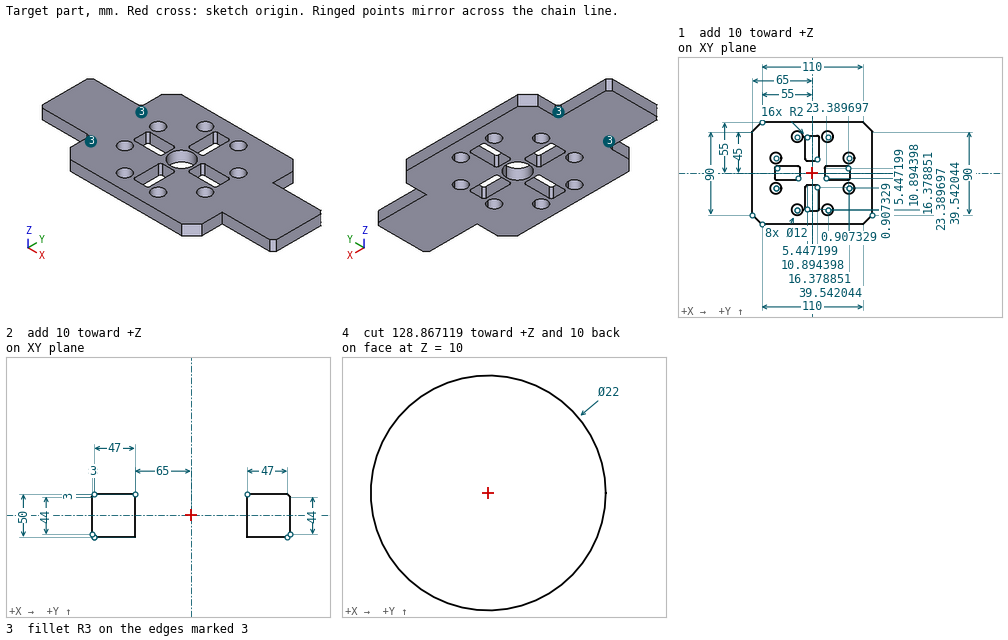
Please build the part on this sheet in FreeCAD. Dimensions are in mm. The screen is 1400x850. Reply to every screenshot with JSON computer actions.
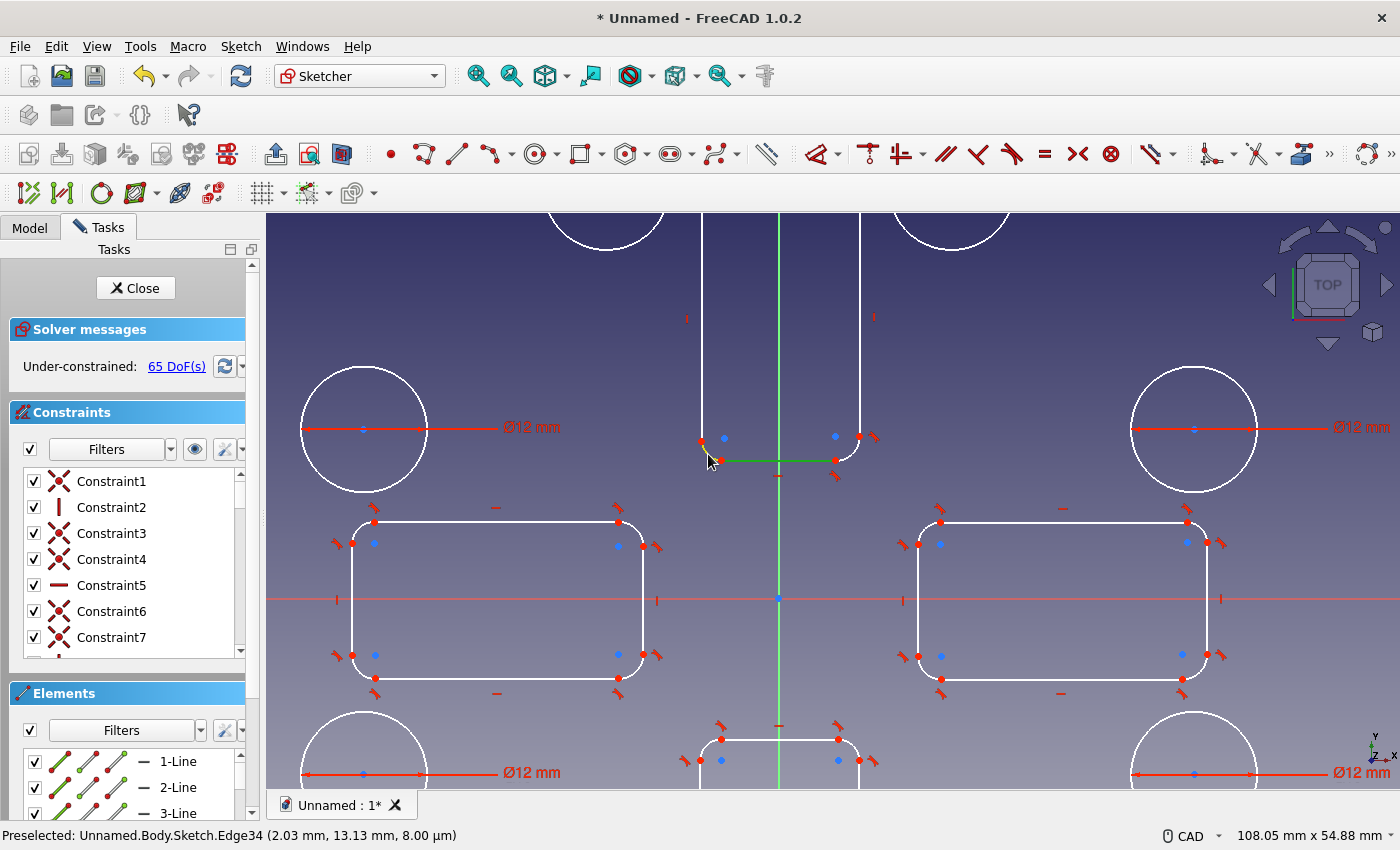
{"action": "left_click", "coordinate": [708, 455]}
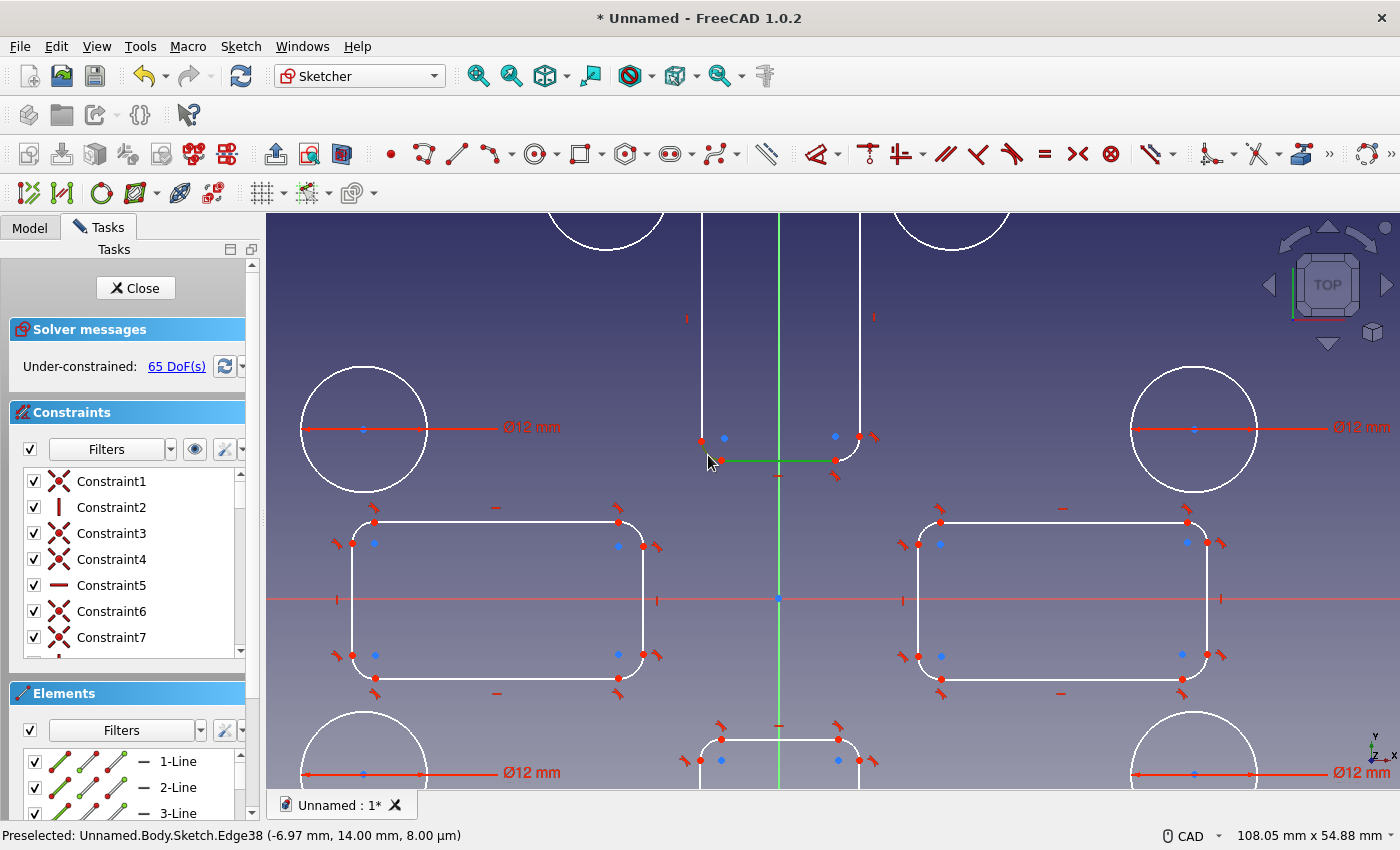
{"action": "left_click", "coordinate": [1012, 154]}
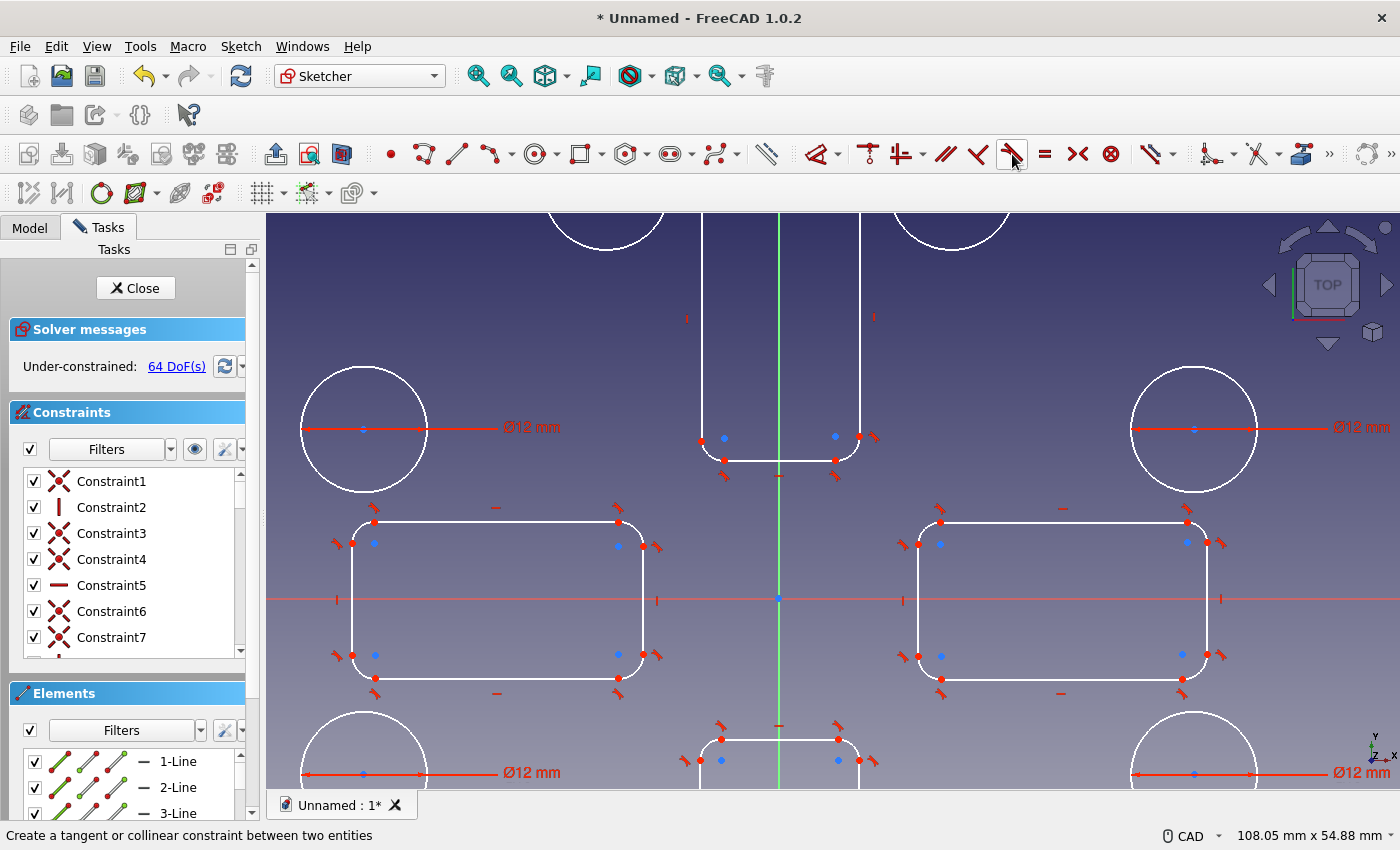
{"action": "left_click", "coordinate": [702, 368]}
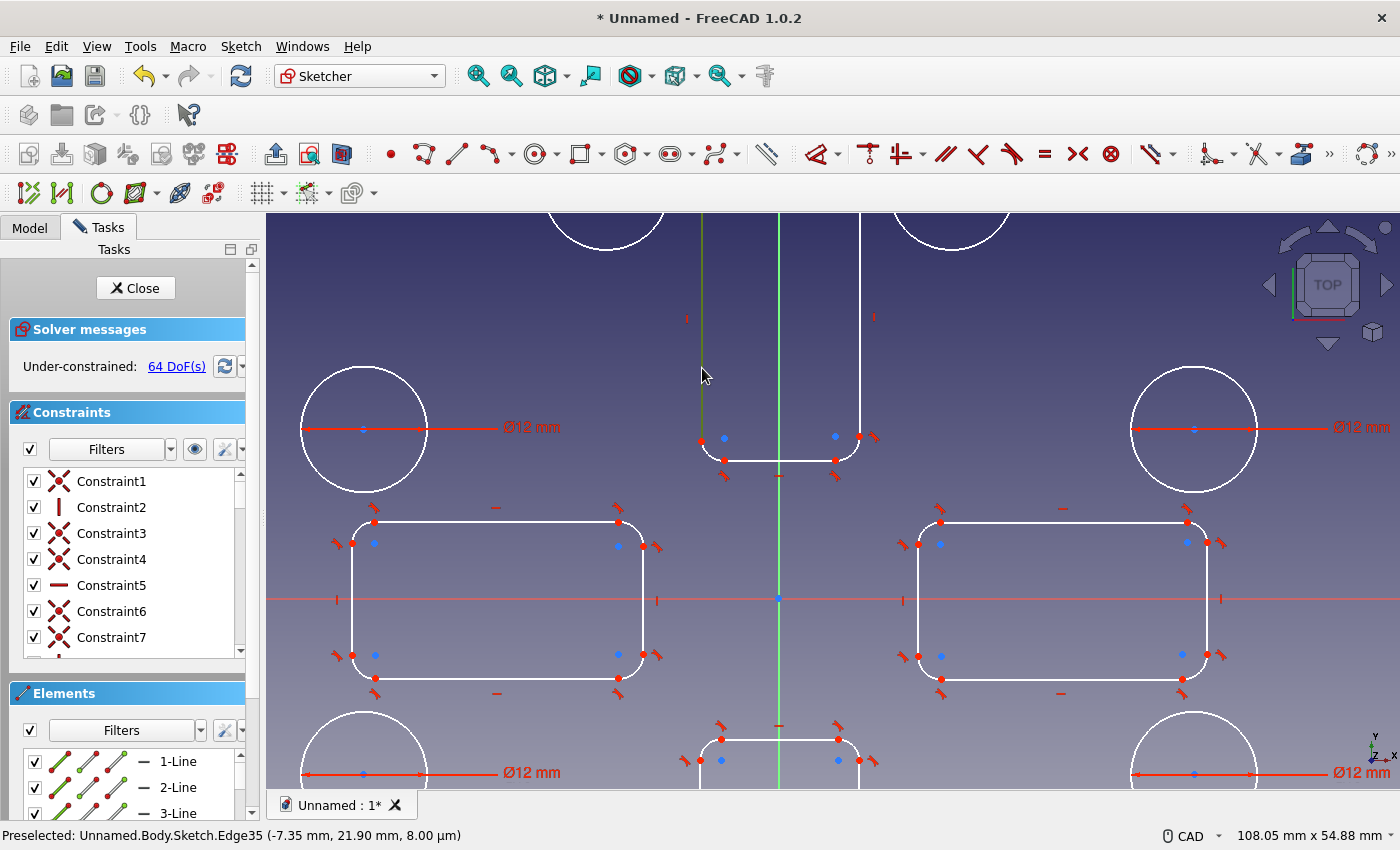
{"action": "scroll", "coordinate": [705, 450], "scroll_direction": "up", "scroll_amount": 2}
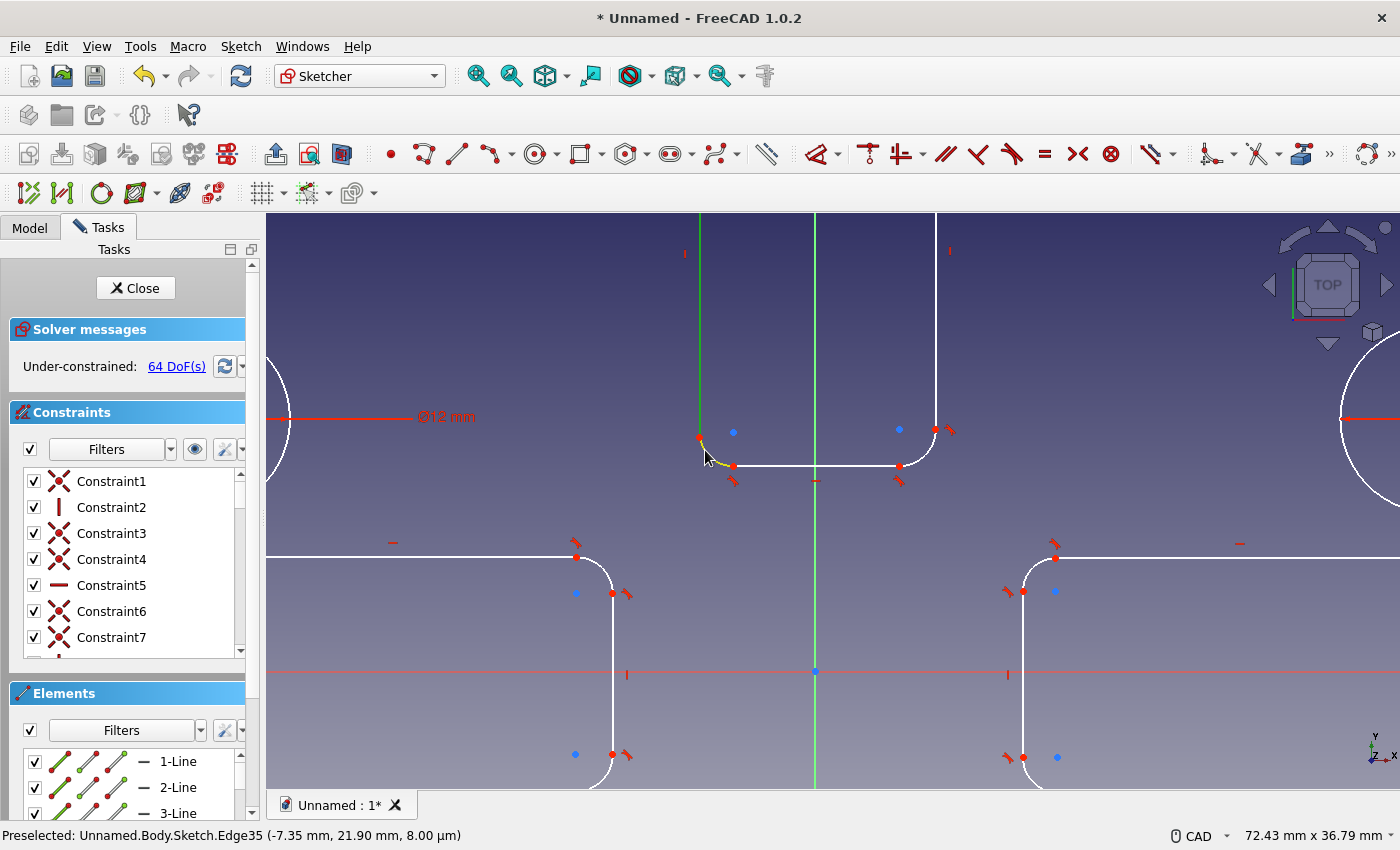
{"action": "left_click", "coordinate": [705, 451]}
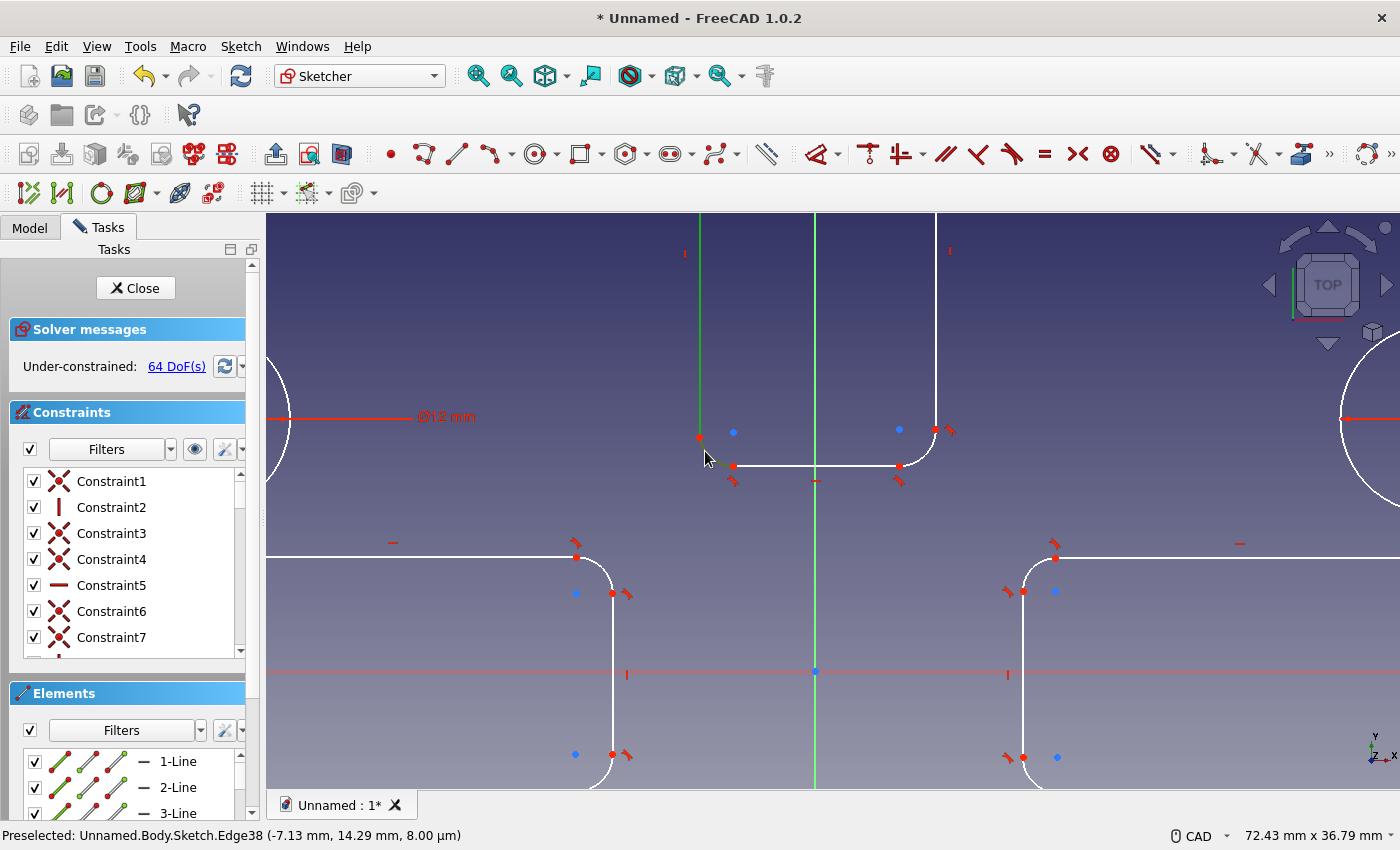
{"action": "left_click", "coordinate": [1012, 154]}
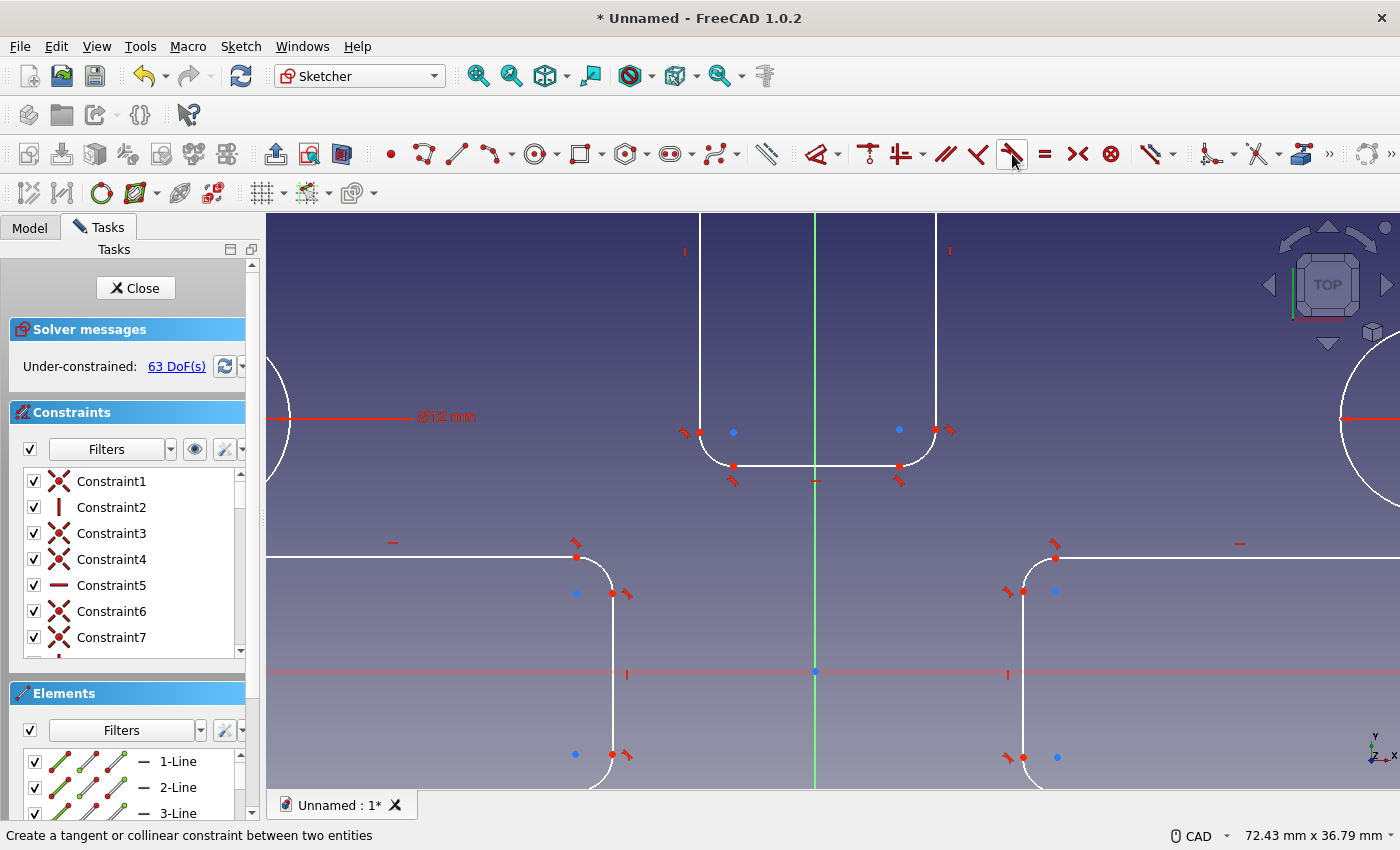
{"action": "scroll", "coordinate": [752, 458], "scroll_direction": "down", "scroll_amount": 8}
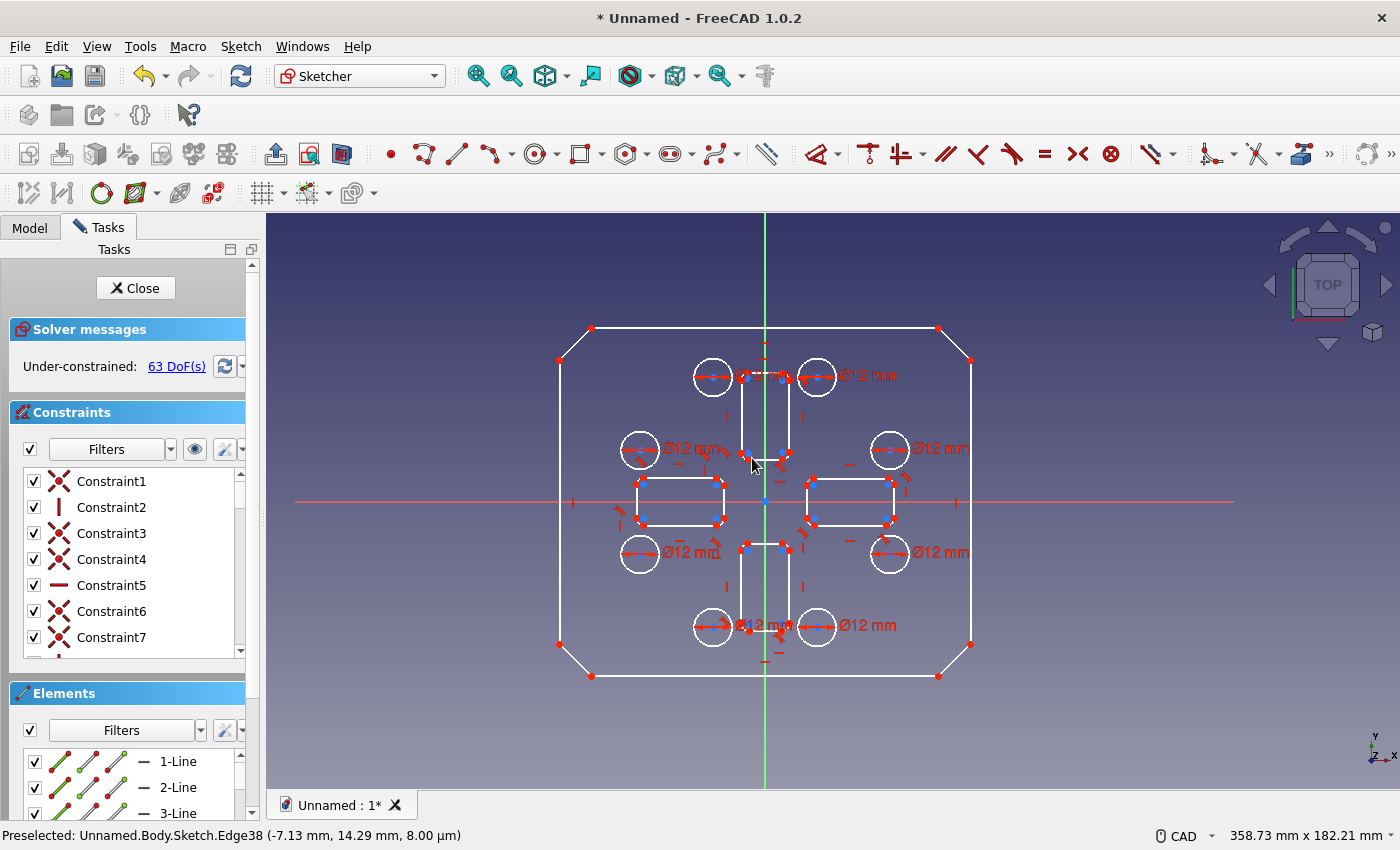
{"action": "left_click", "coordinate": [742, 431]}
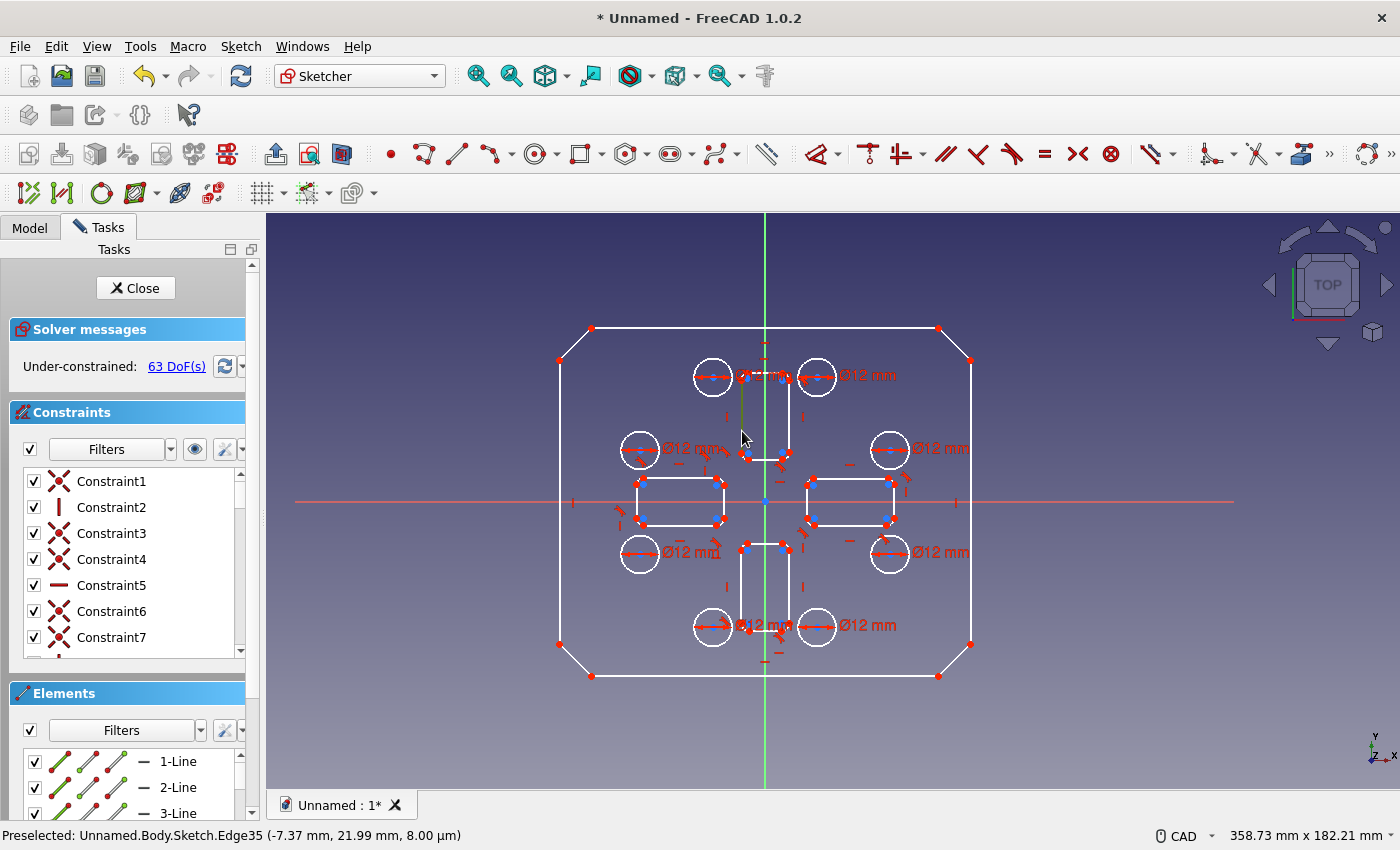
{"action": "scroll", "coordinate": [743, 375], "scroll_direction": "up", "scroll_amount": 5}